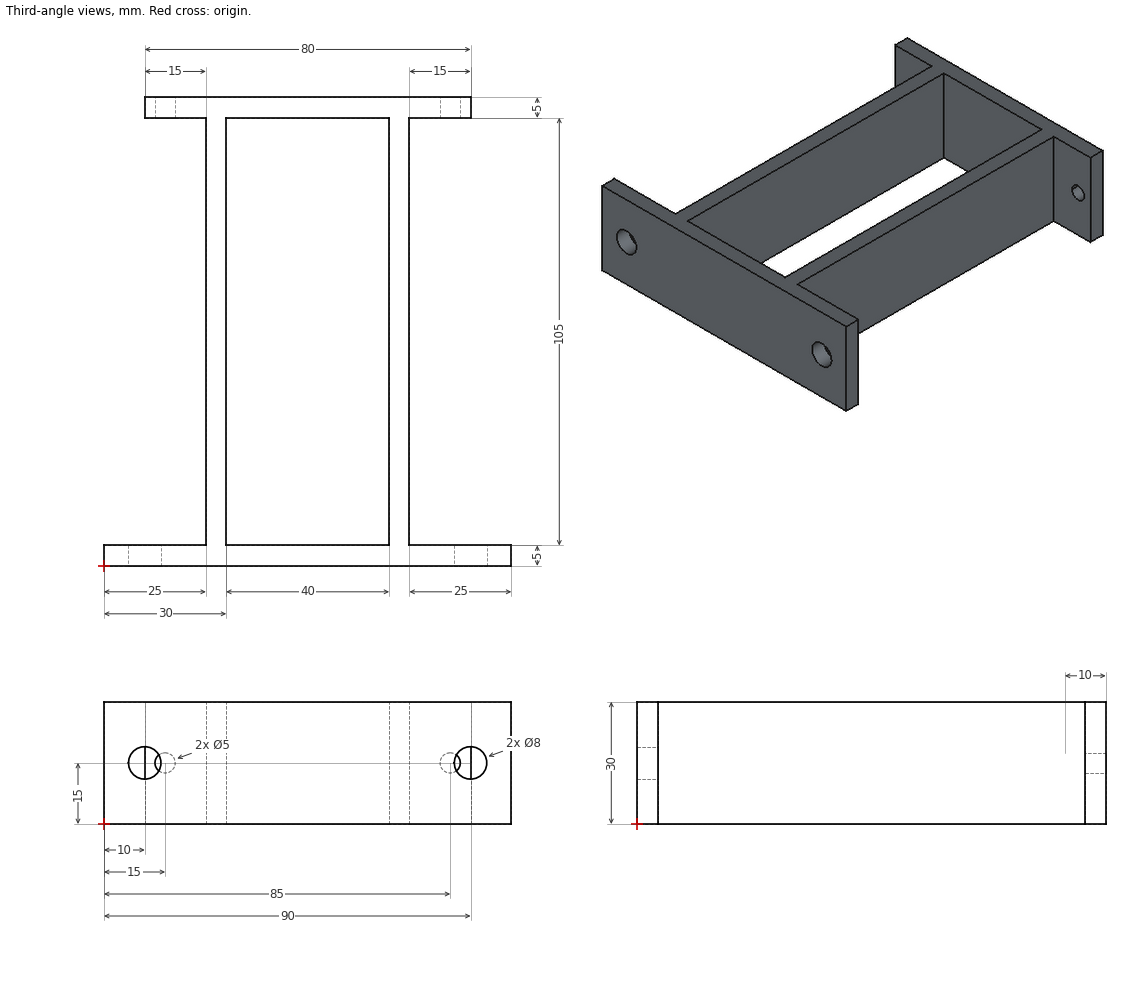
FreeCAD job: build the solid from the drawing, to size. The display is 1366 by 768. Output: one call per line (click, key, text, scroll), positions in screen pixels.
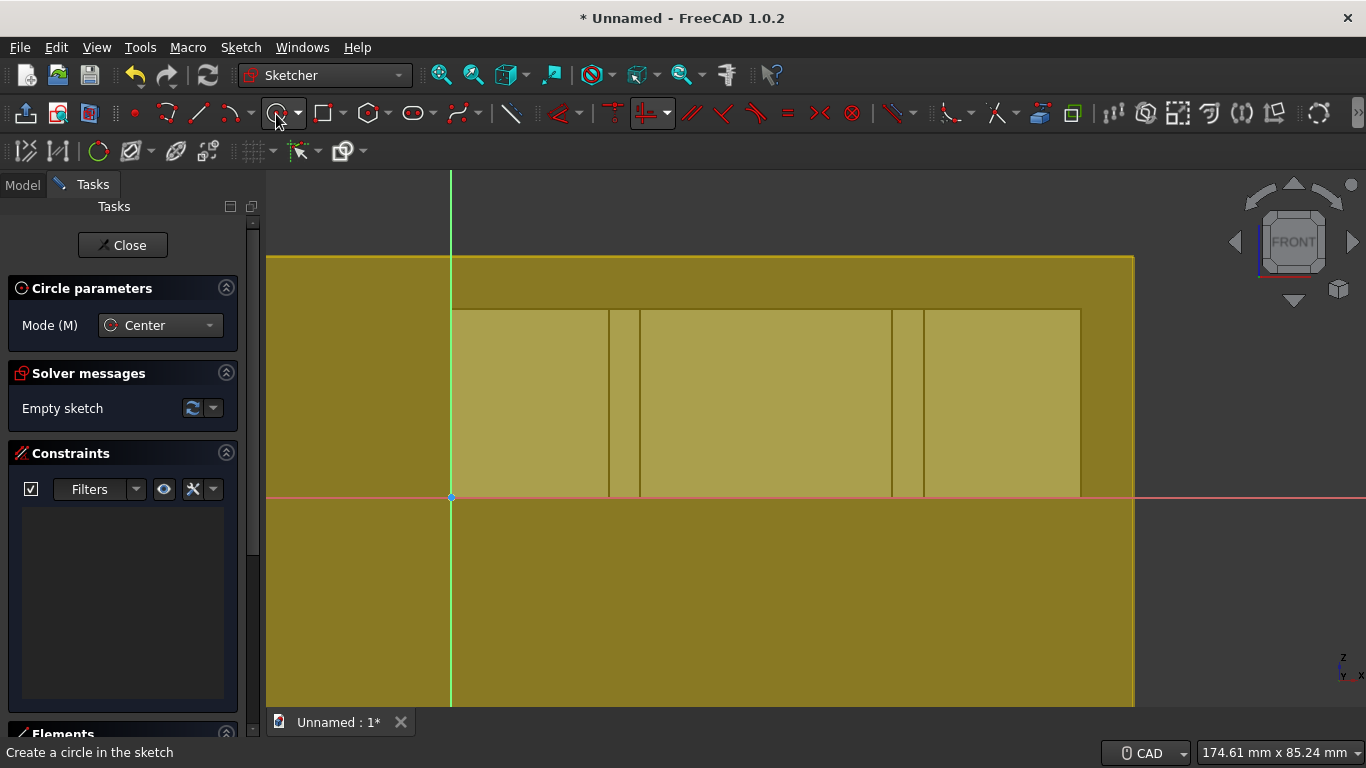
click(1018, 403)
click(1036, 385)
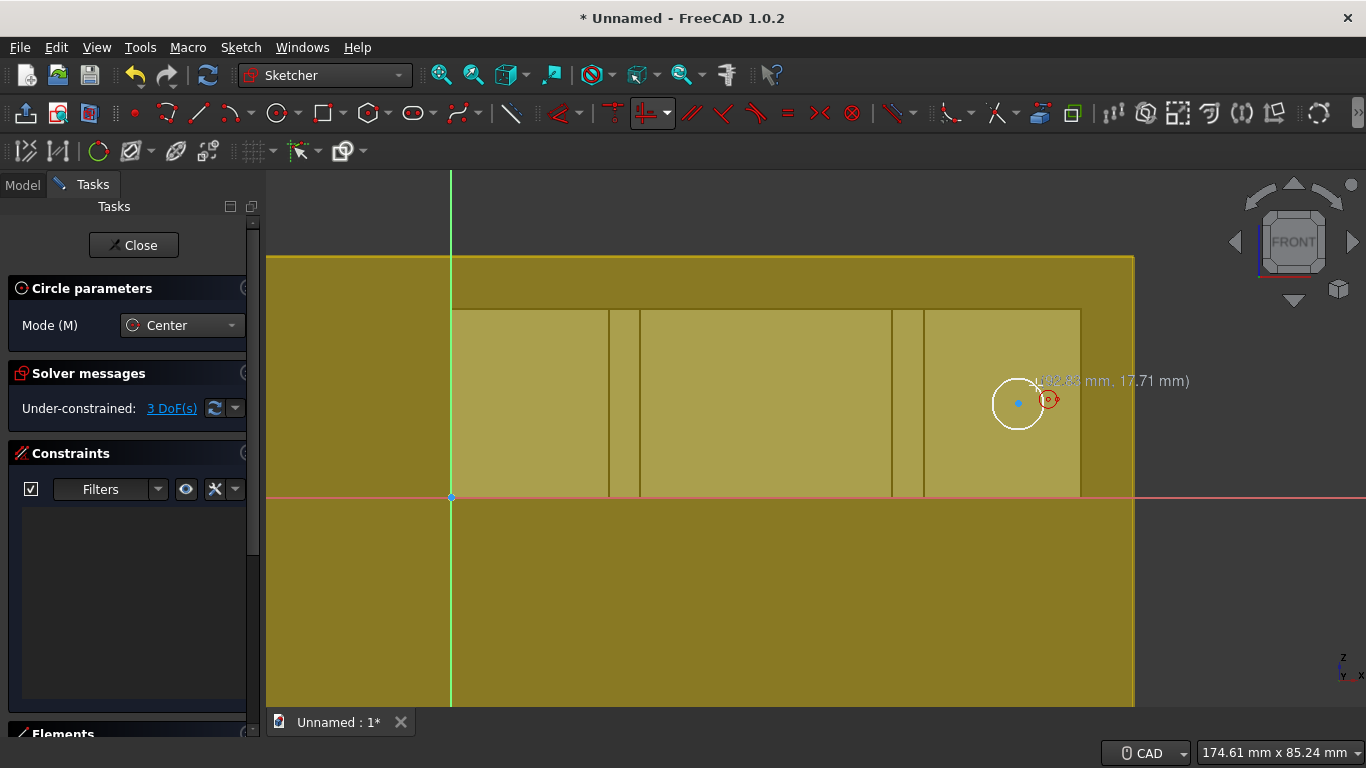
click(514, 403)
click(532, 385)
key(Escape)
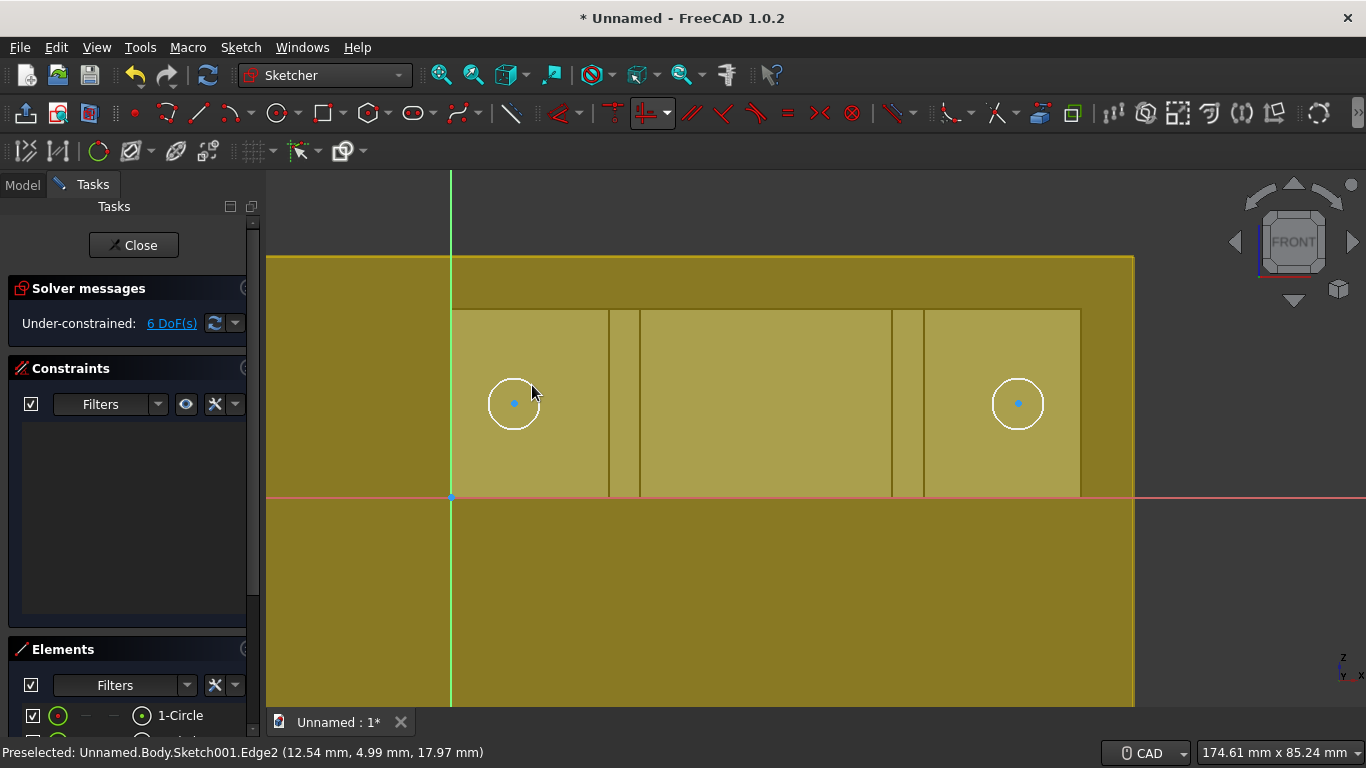
click(1036, 386)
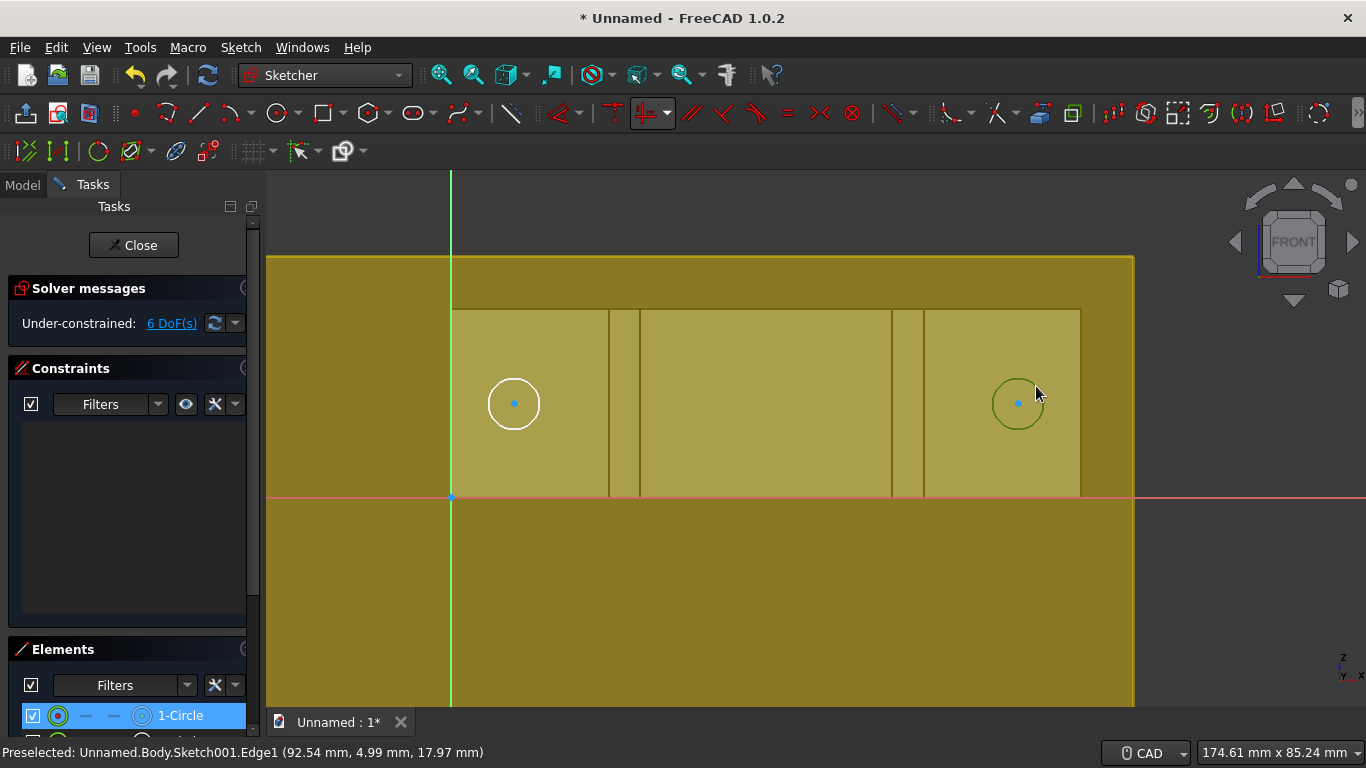
click(532, 386)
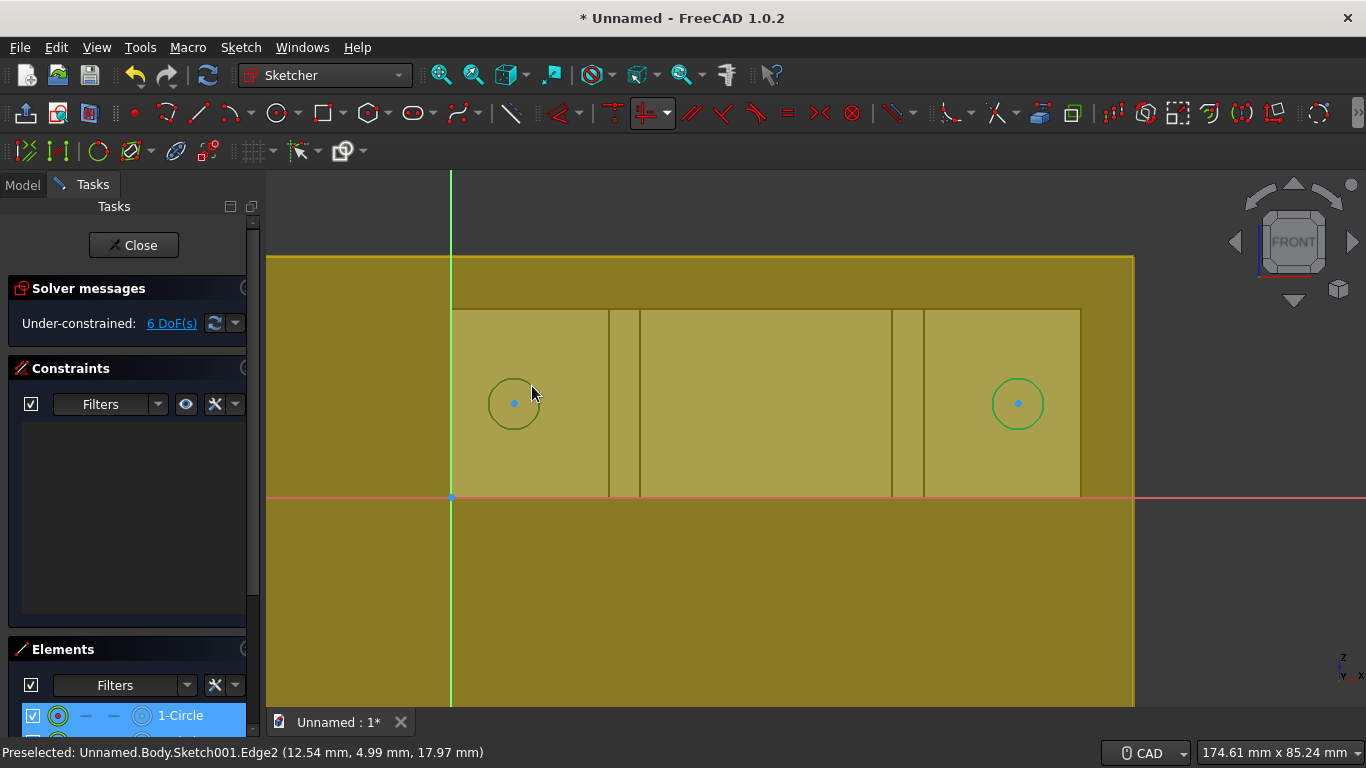
click(788, 114)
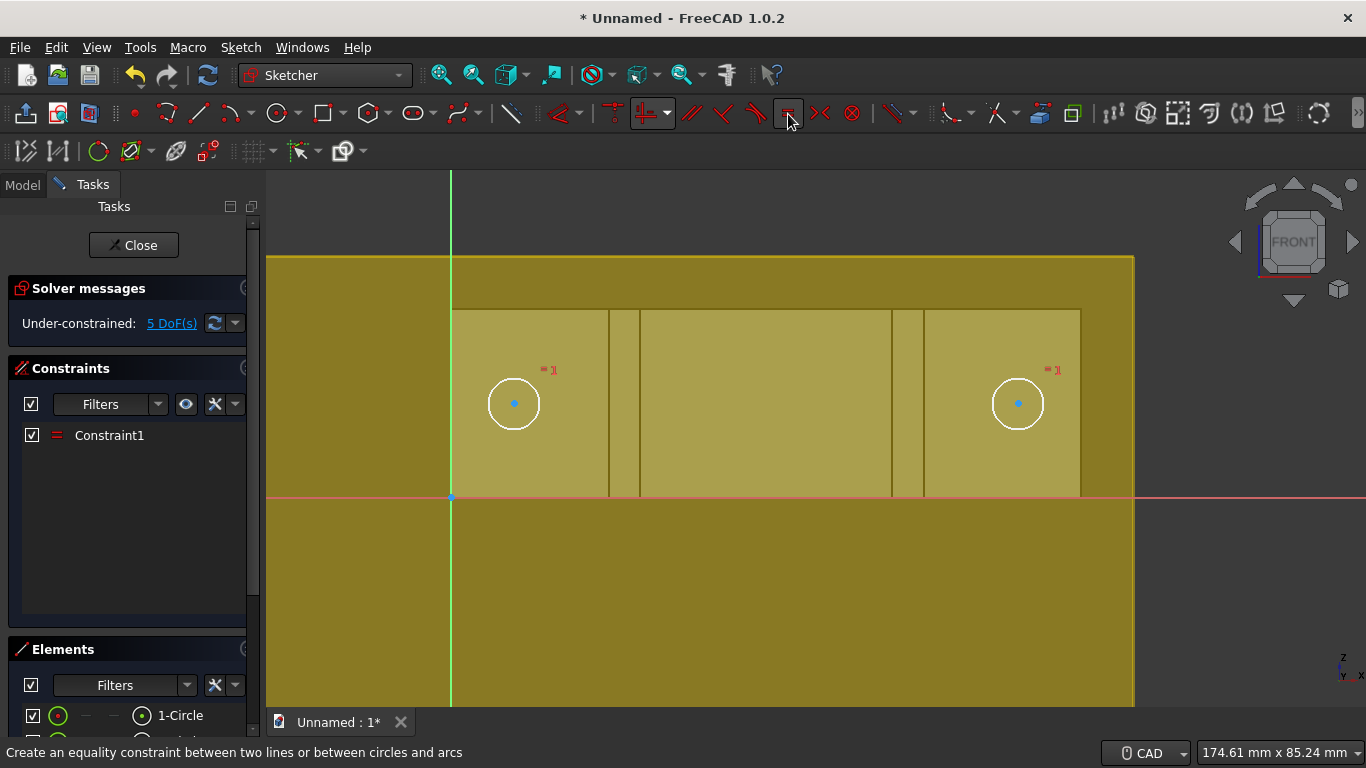
click(1018, 404)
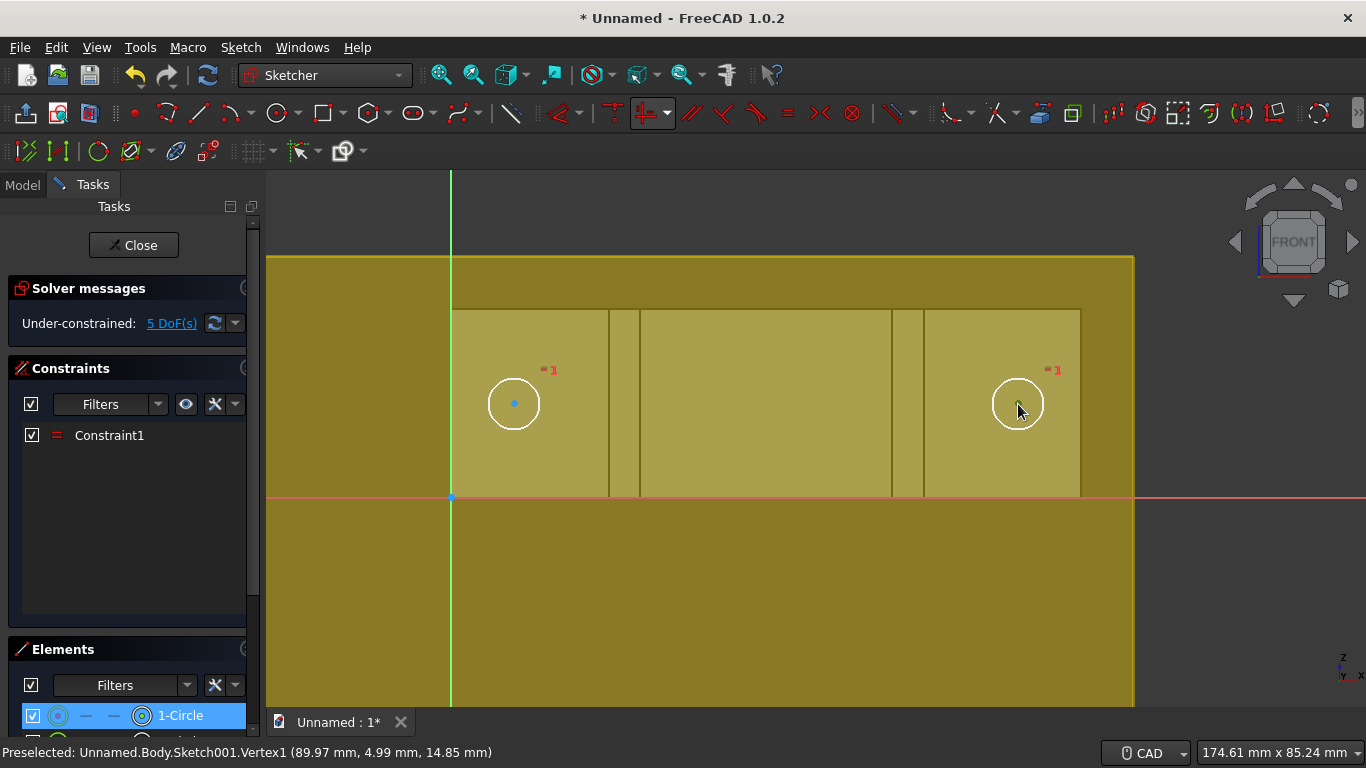
click(514, 404)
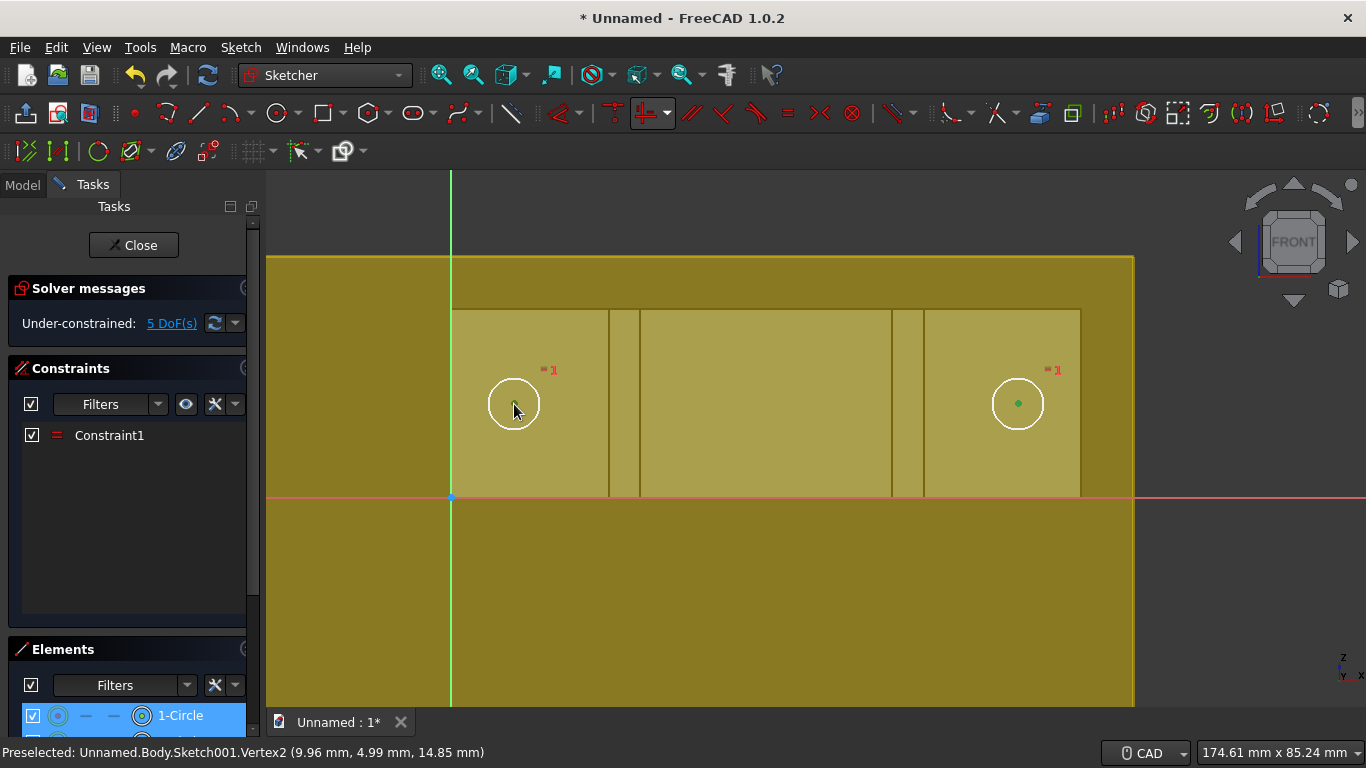
click(670, 114)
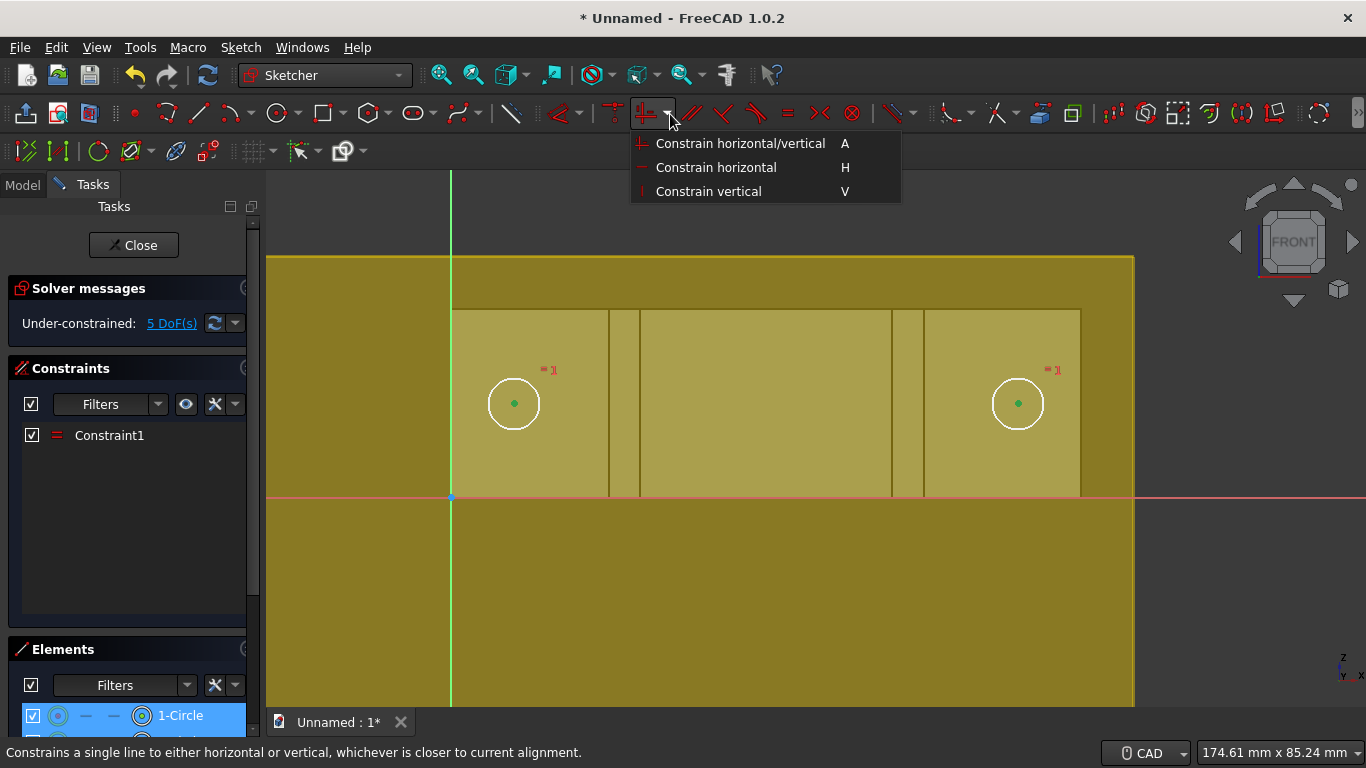
click(766, 167)